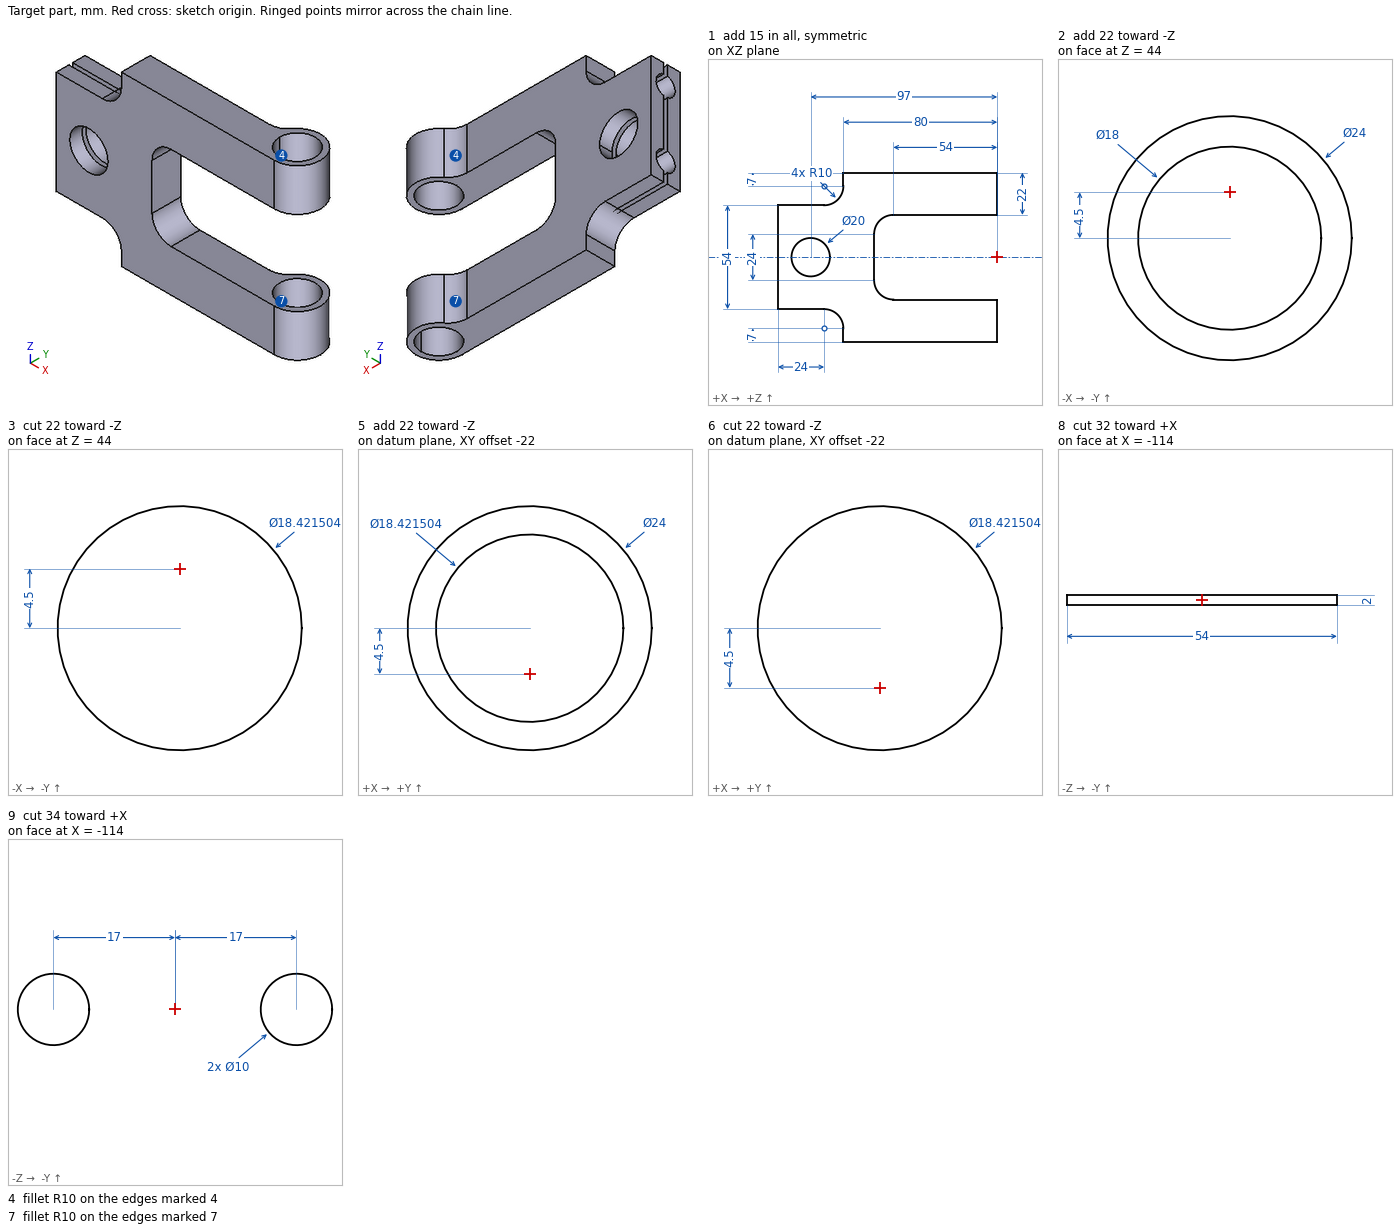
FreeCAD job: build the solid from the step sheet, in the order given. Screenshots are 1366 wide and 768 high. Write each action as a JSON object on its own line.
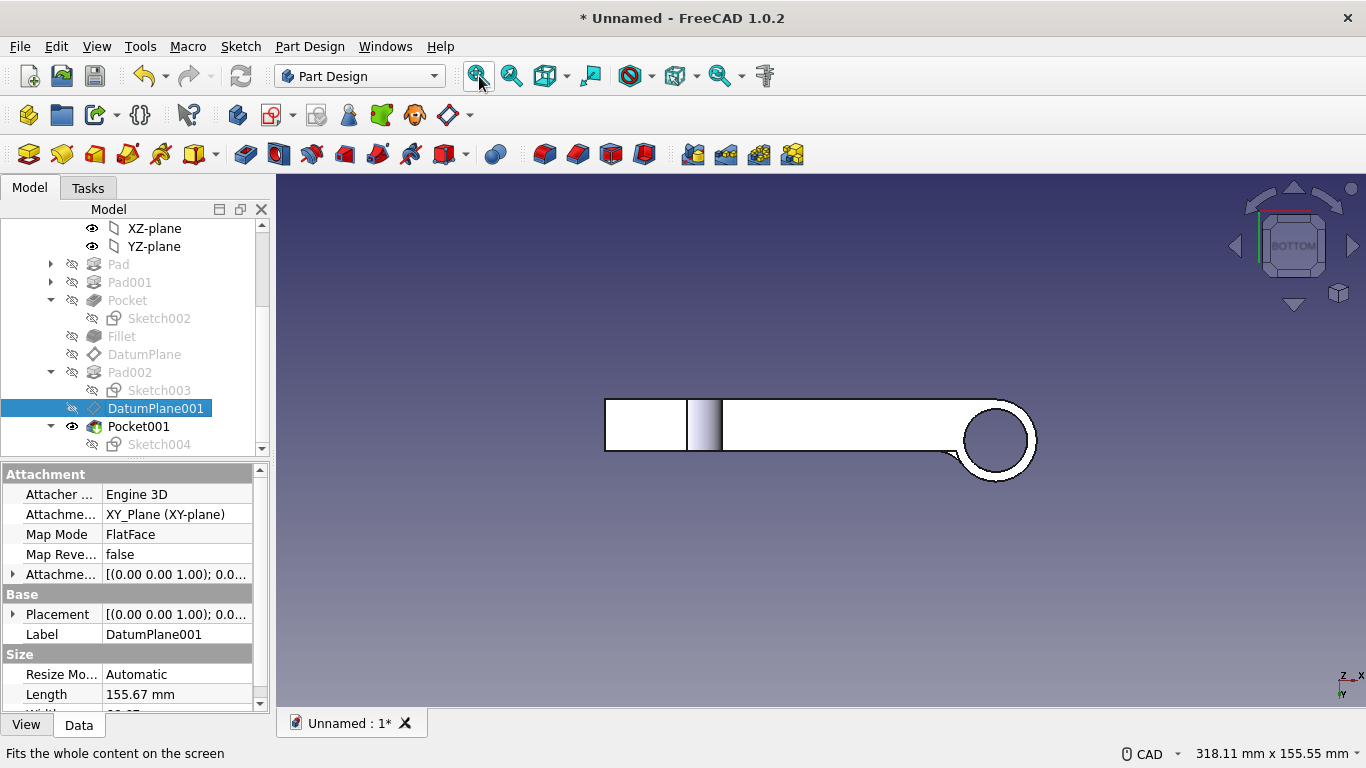
{"action": "left_click", "coordinate": [479, 76]}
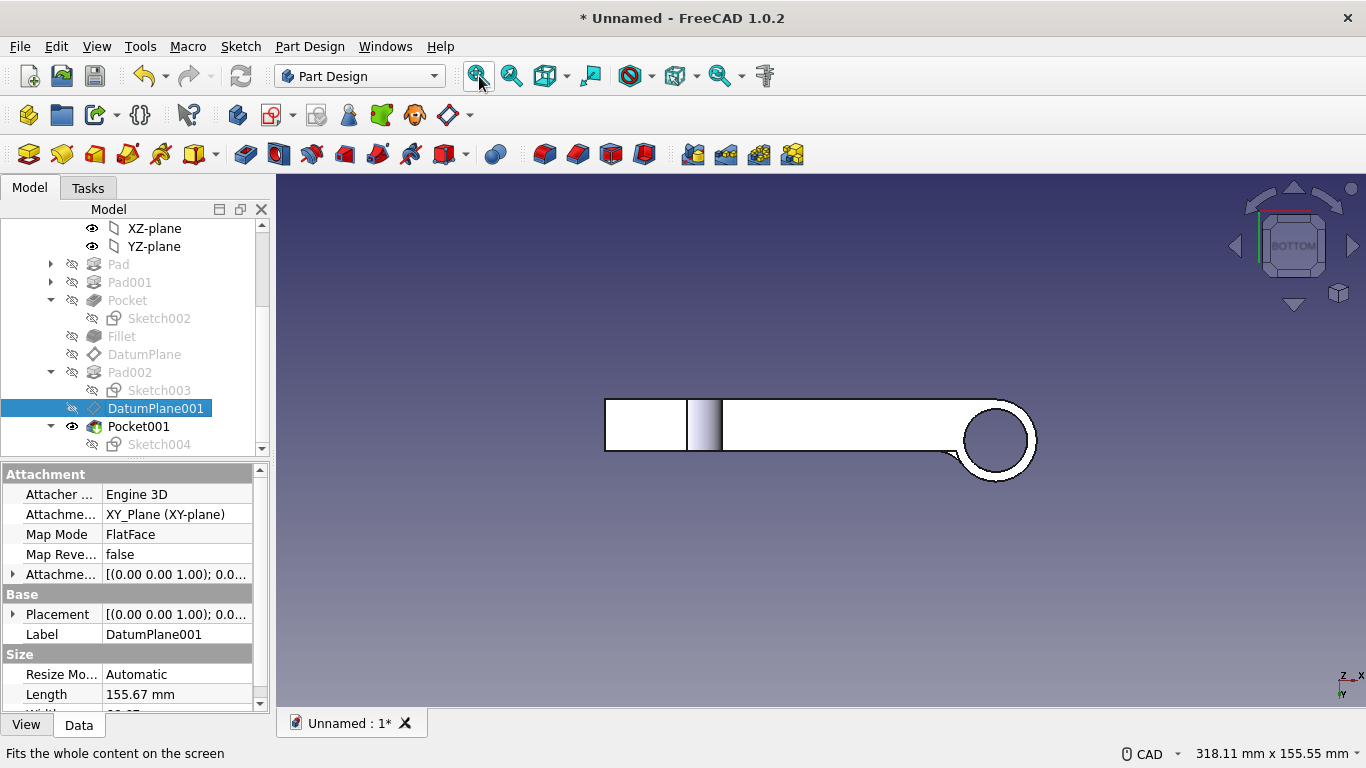
{"action": "key", "text": "4"}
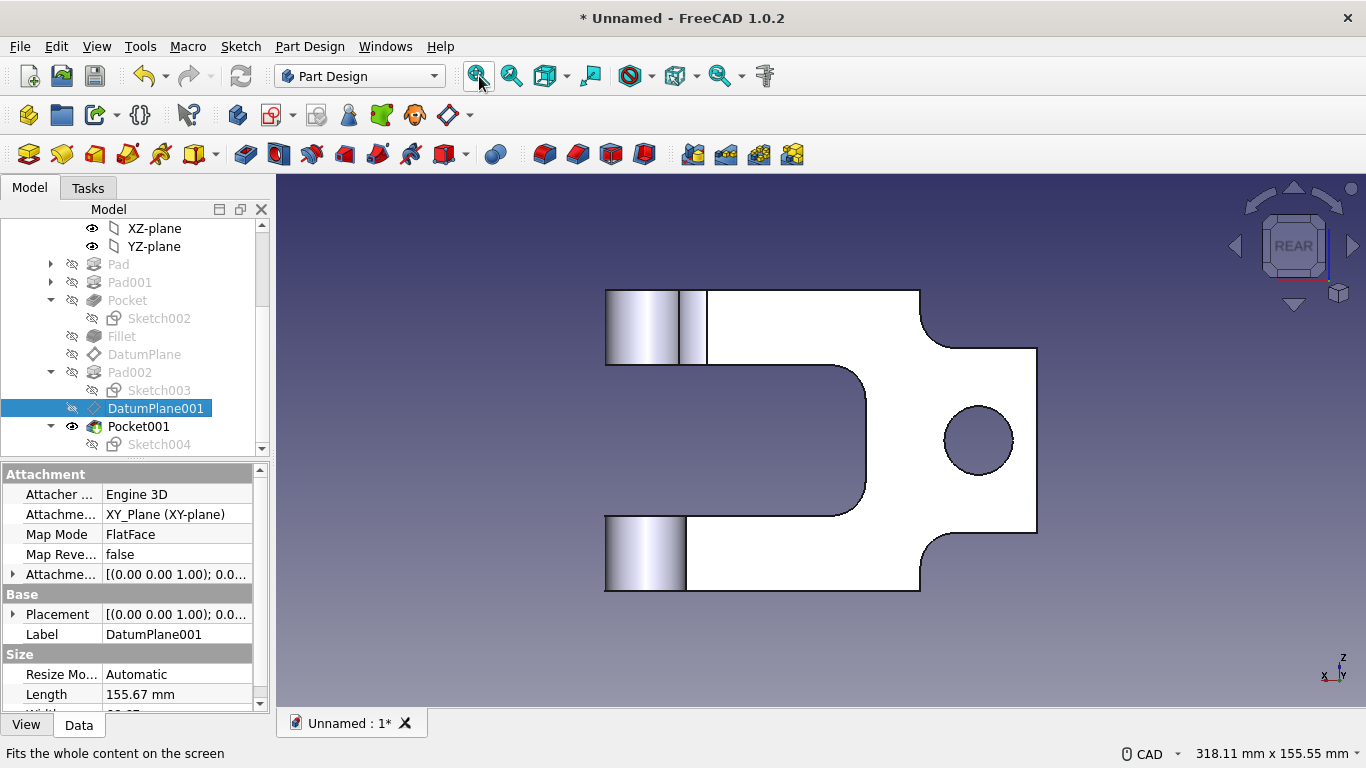
{"action": "key", "text": "6"}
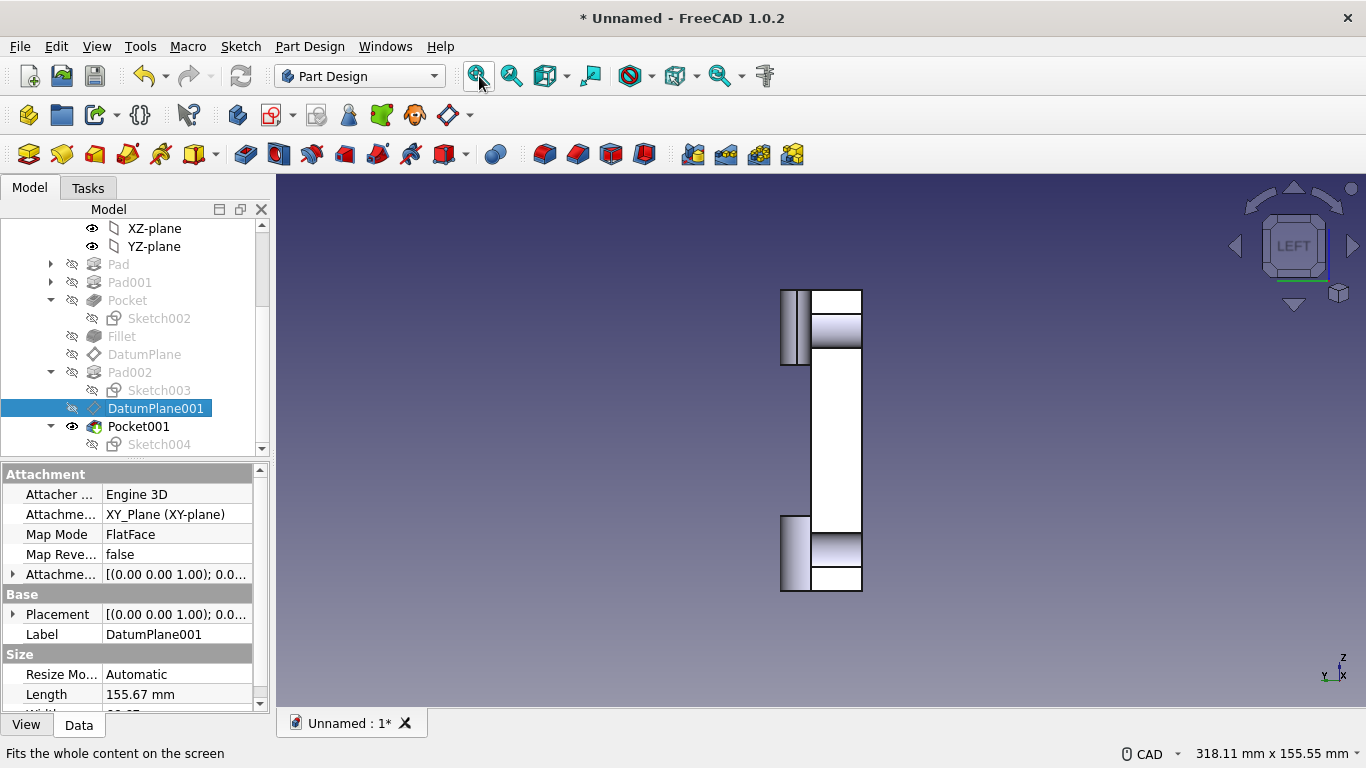
{"action": "key", "text": "v 3"}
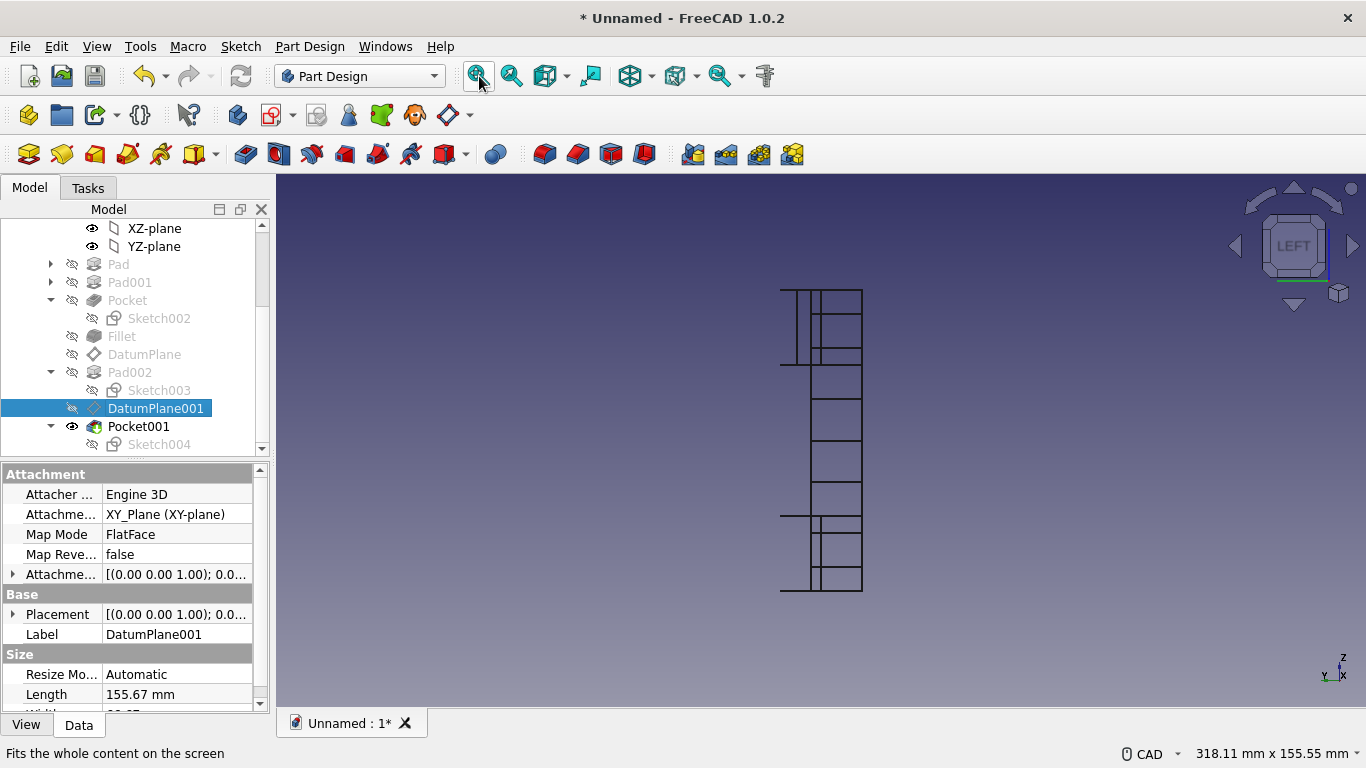
{"action": "key", "text": "0"}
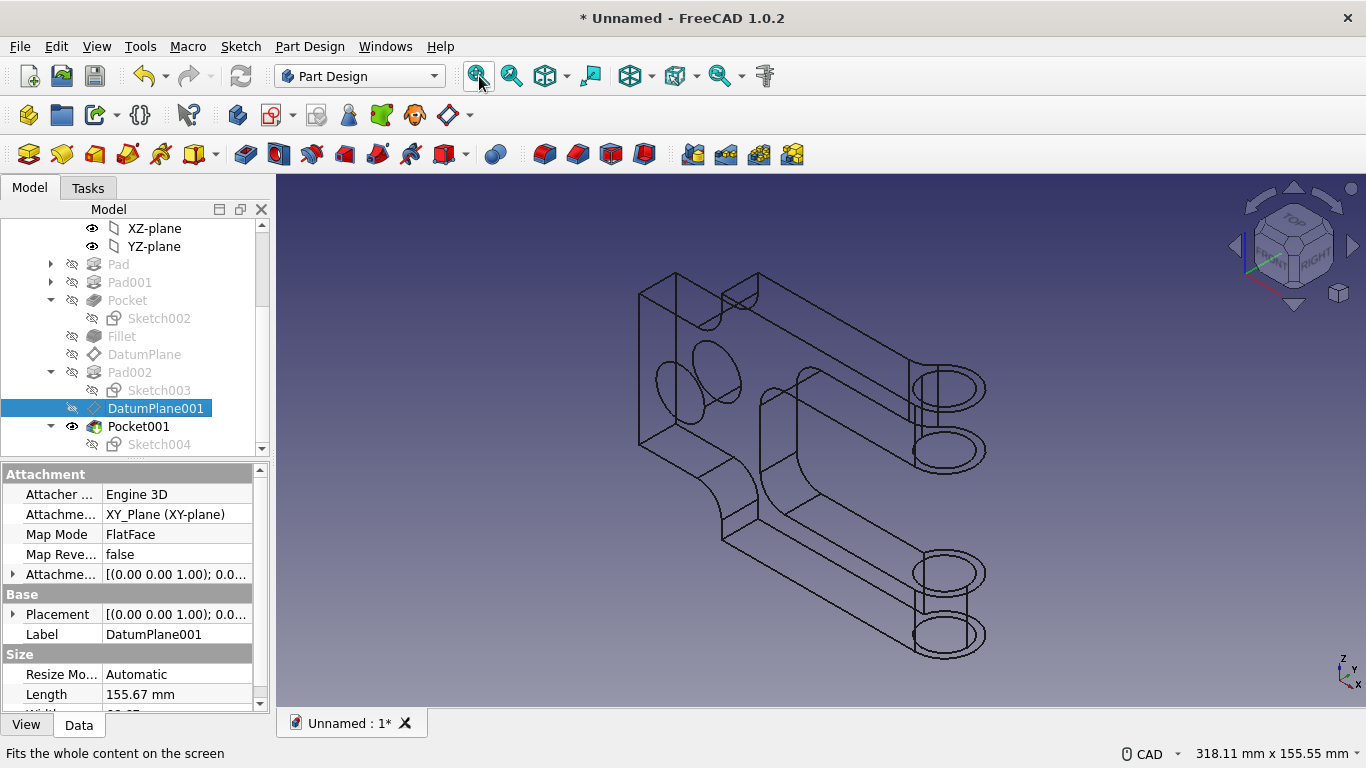
{"action": "left_click", "coordinate": [924, 577]}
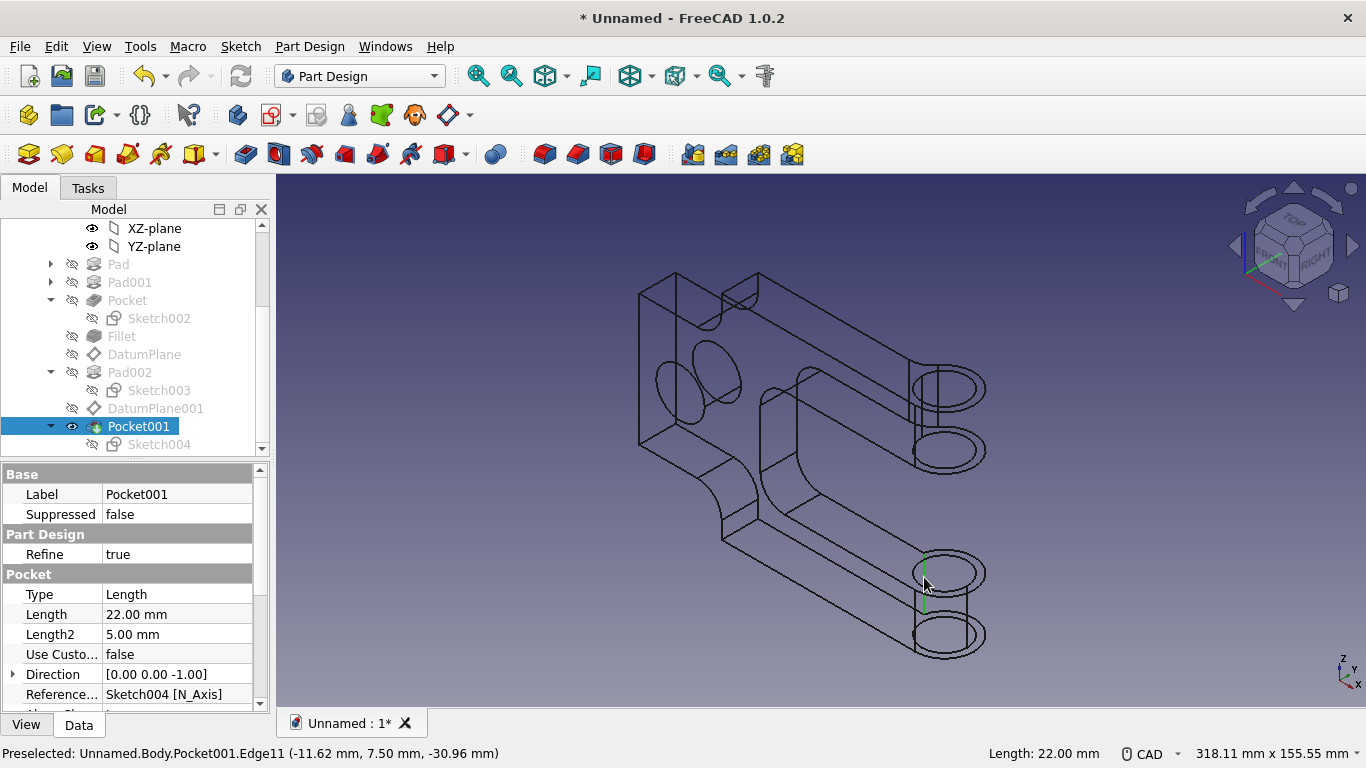
{"action": "key", "text": "v 1"}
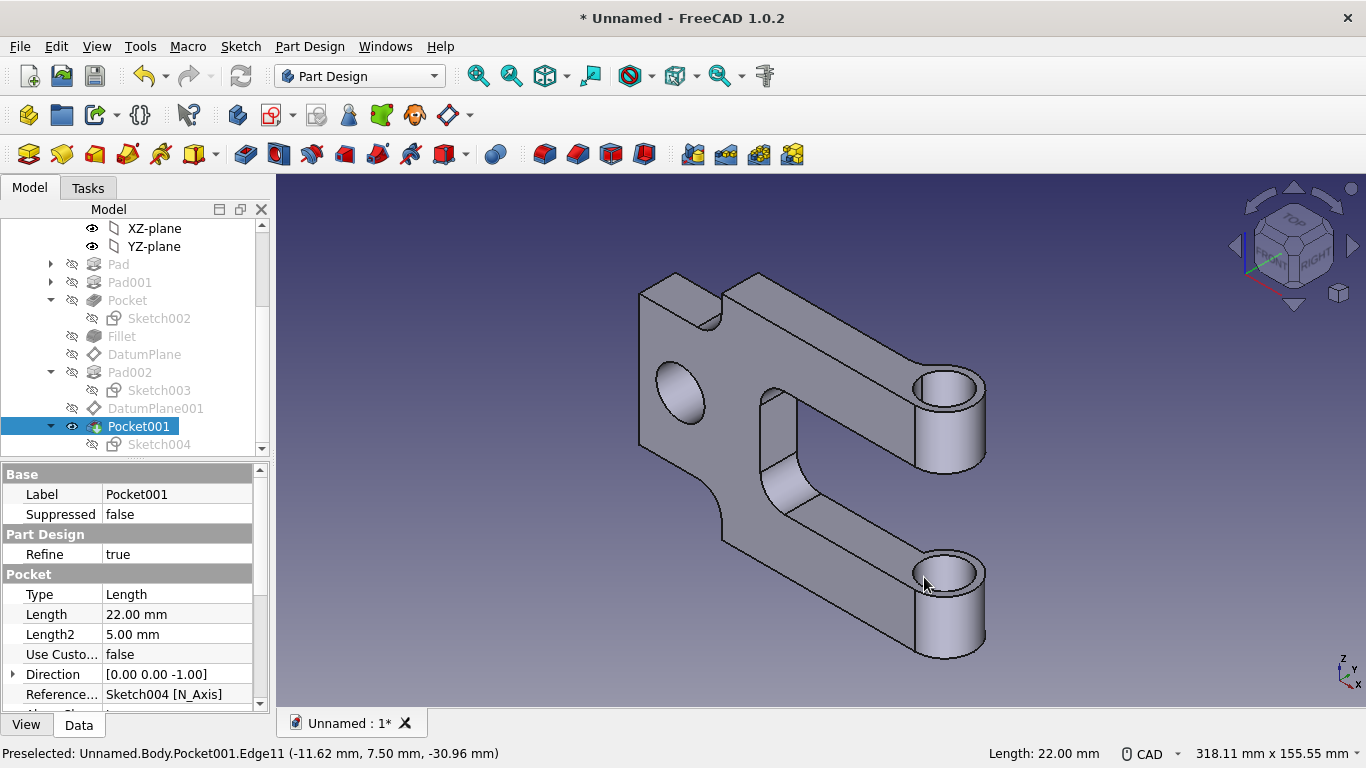
{"action": "left_click", "coordinate": [545, 154]}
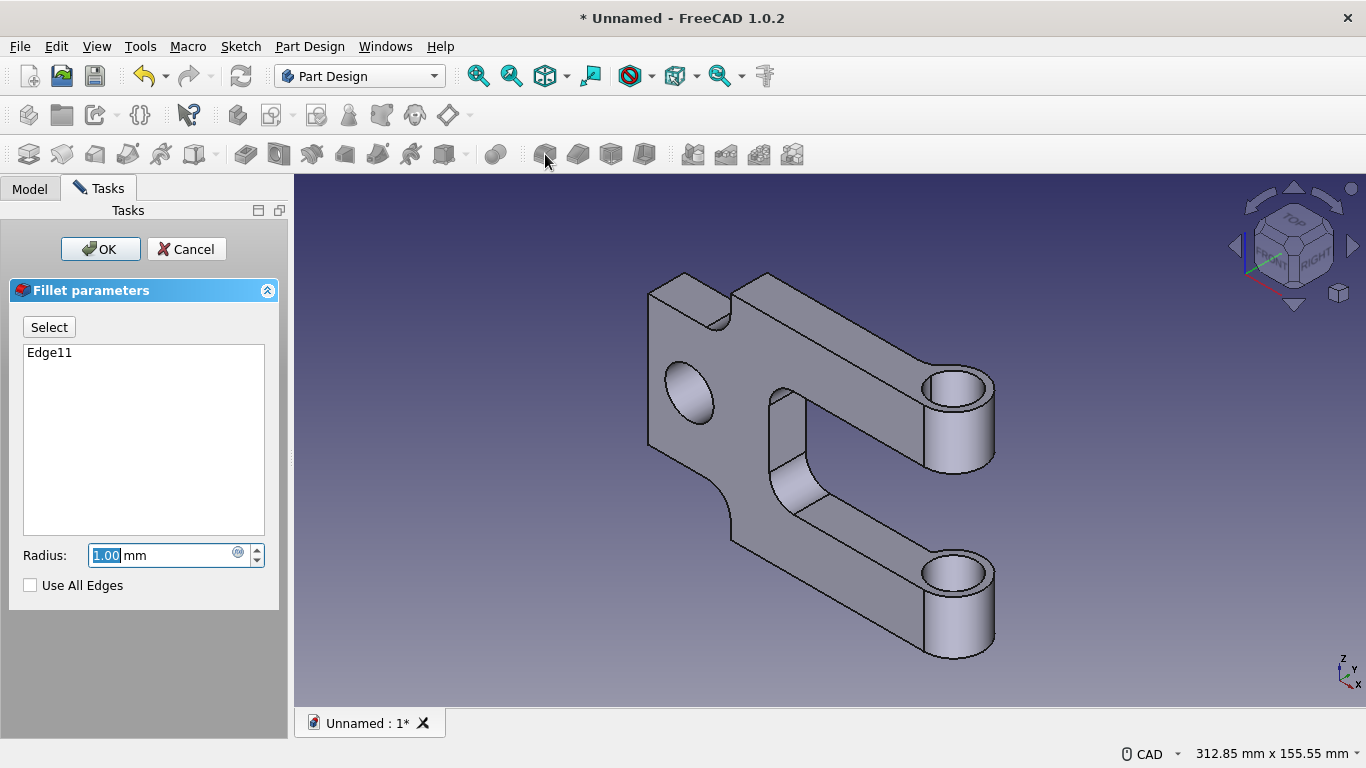
{"action": "type", "text": "10"}
{"action": "key", "text": "Tab"}